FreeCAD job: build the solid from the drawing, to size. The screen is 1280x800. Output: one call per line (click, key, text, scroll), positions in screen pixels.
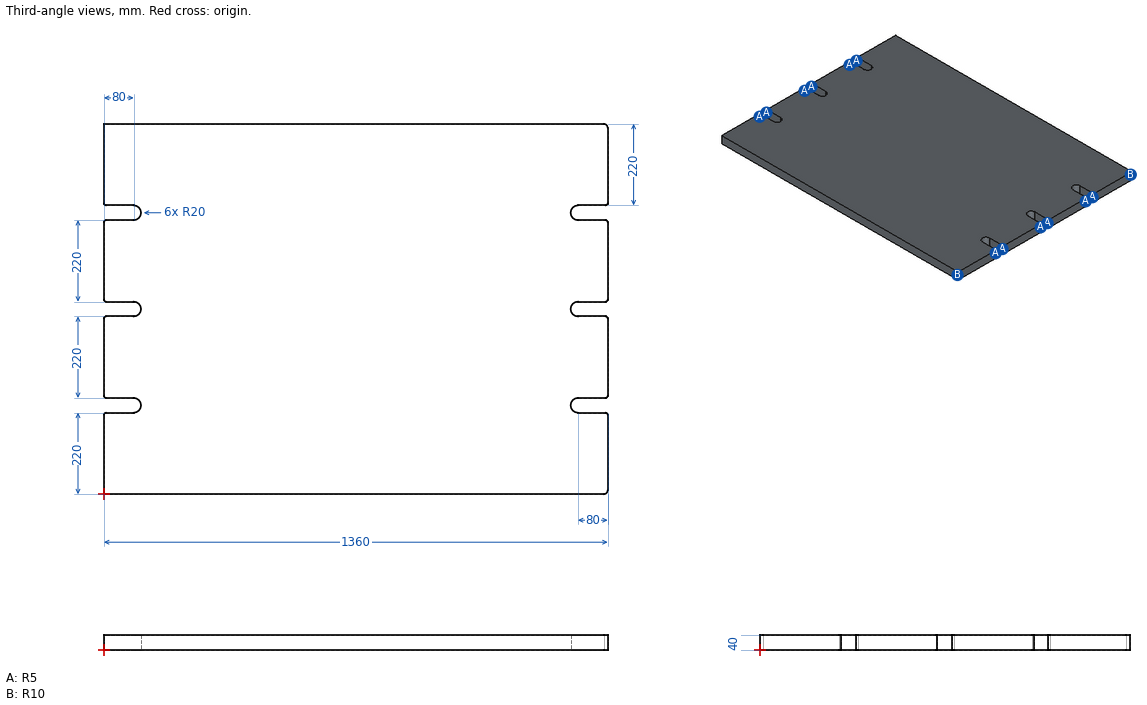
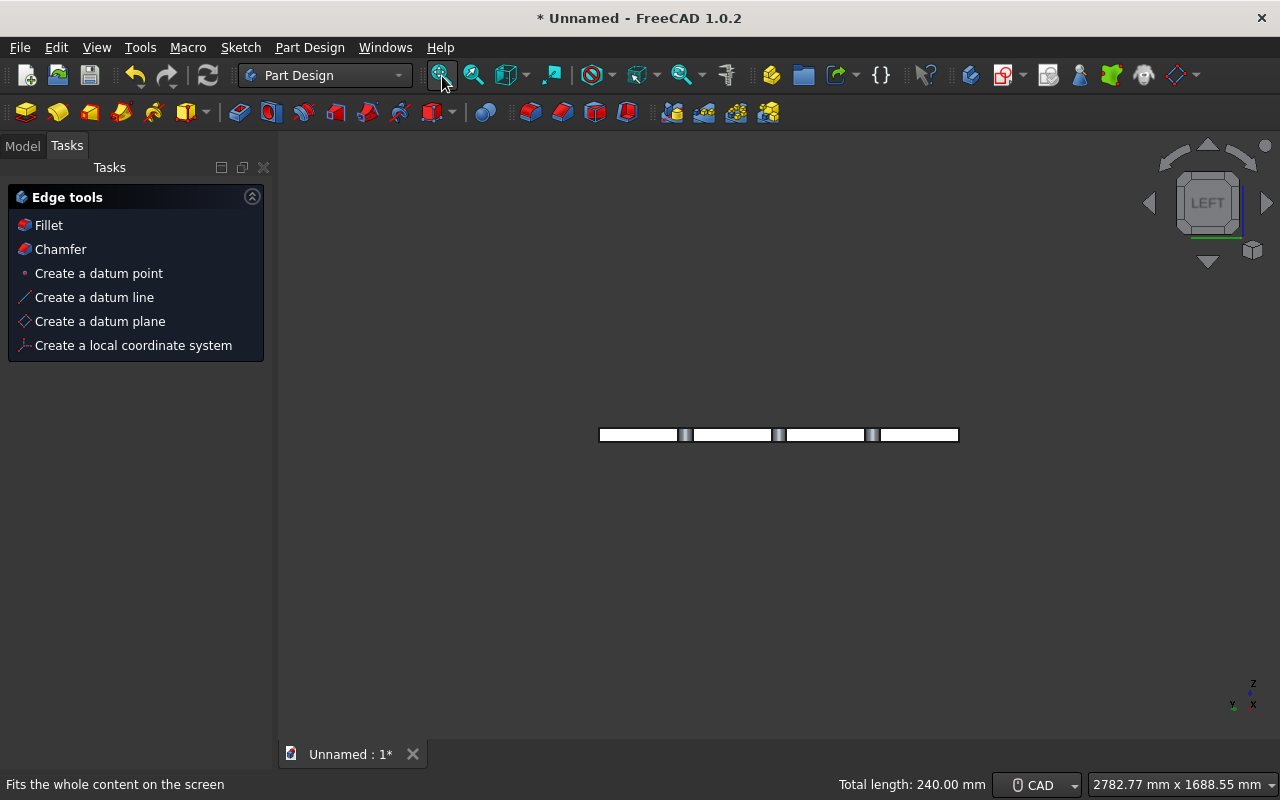
click(880, 434, ctrl)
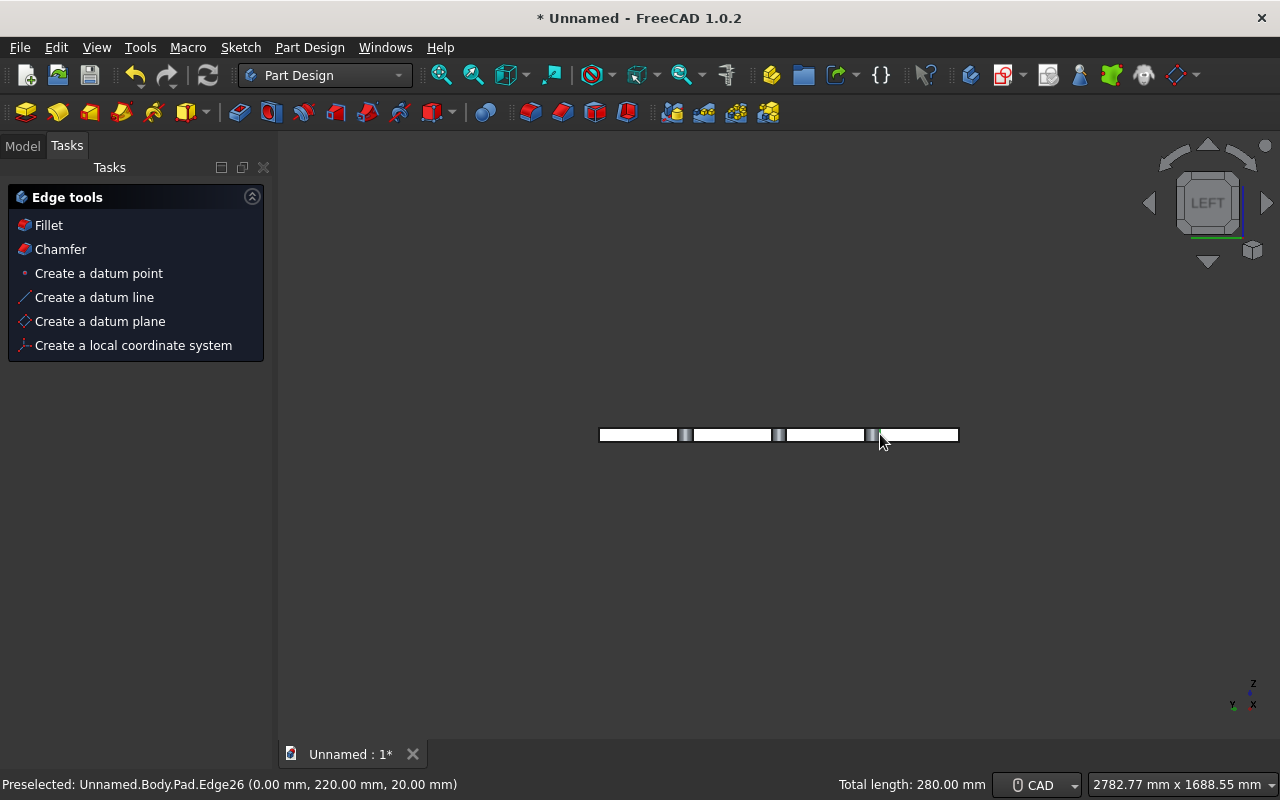
click(865, 434, ctrl)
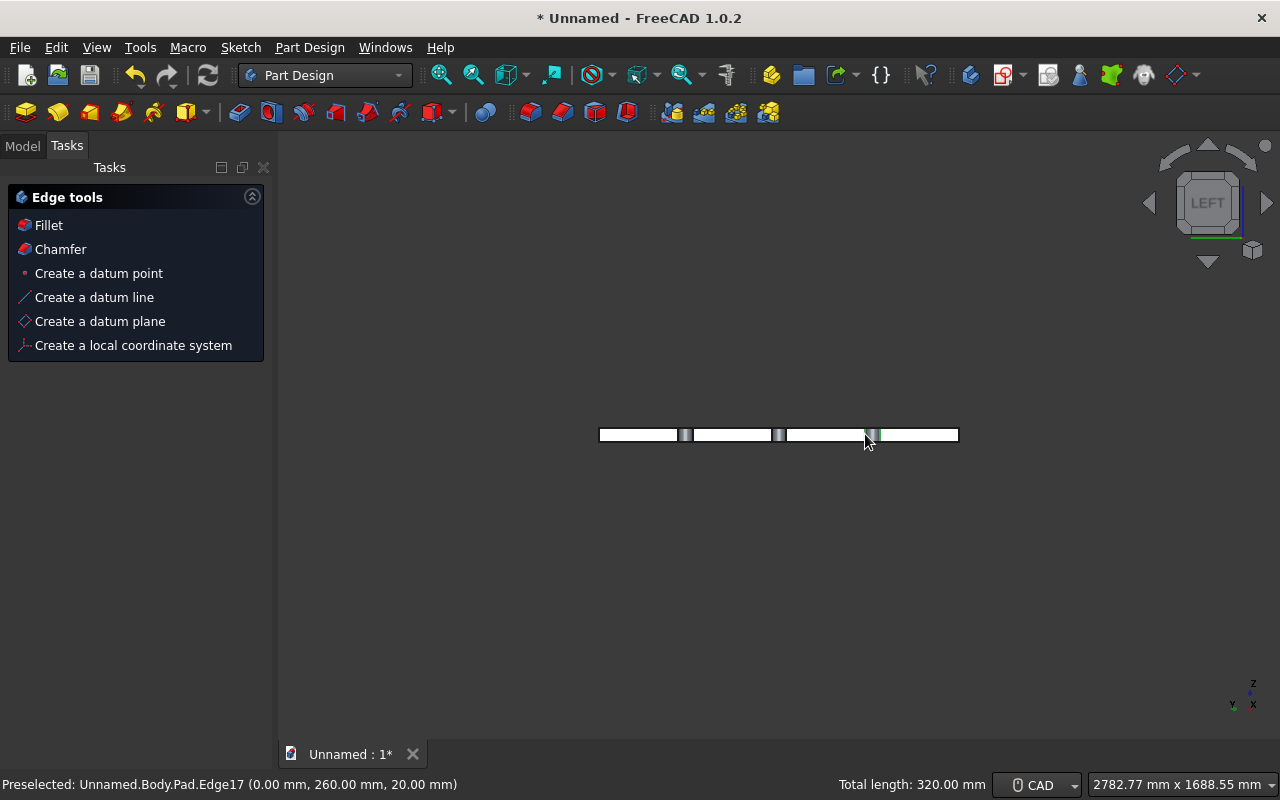
click(786, 434, ctrl)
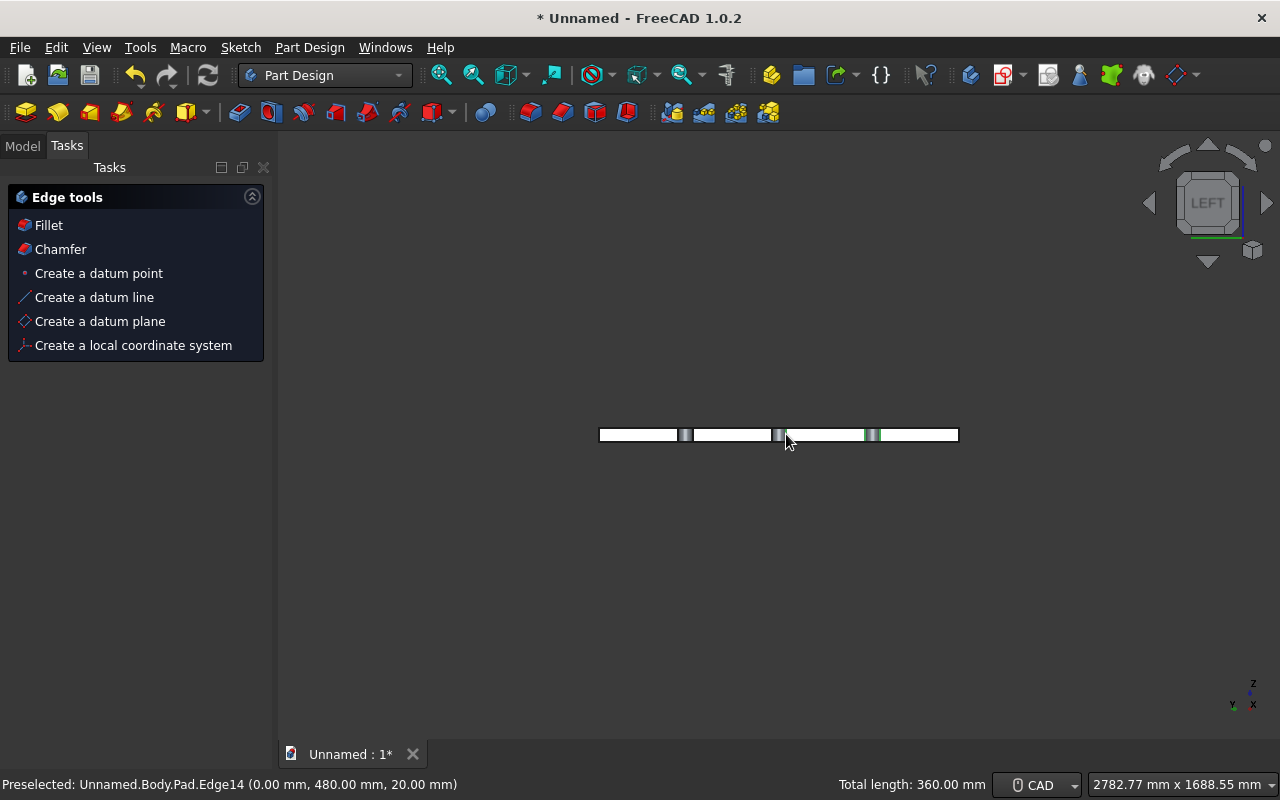
click(772, 434, ctrl)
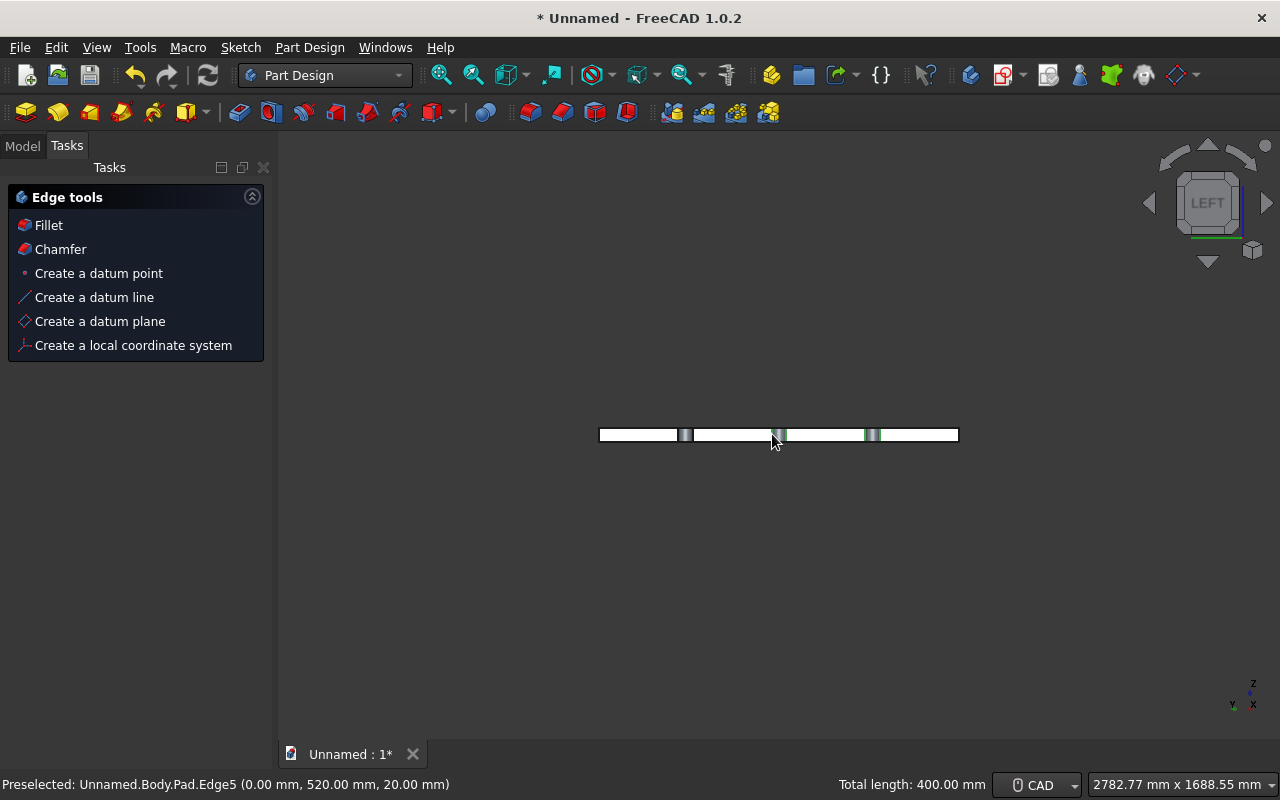
click(693, 434, ctrl)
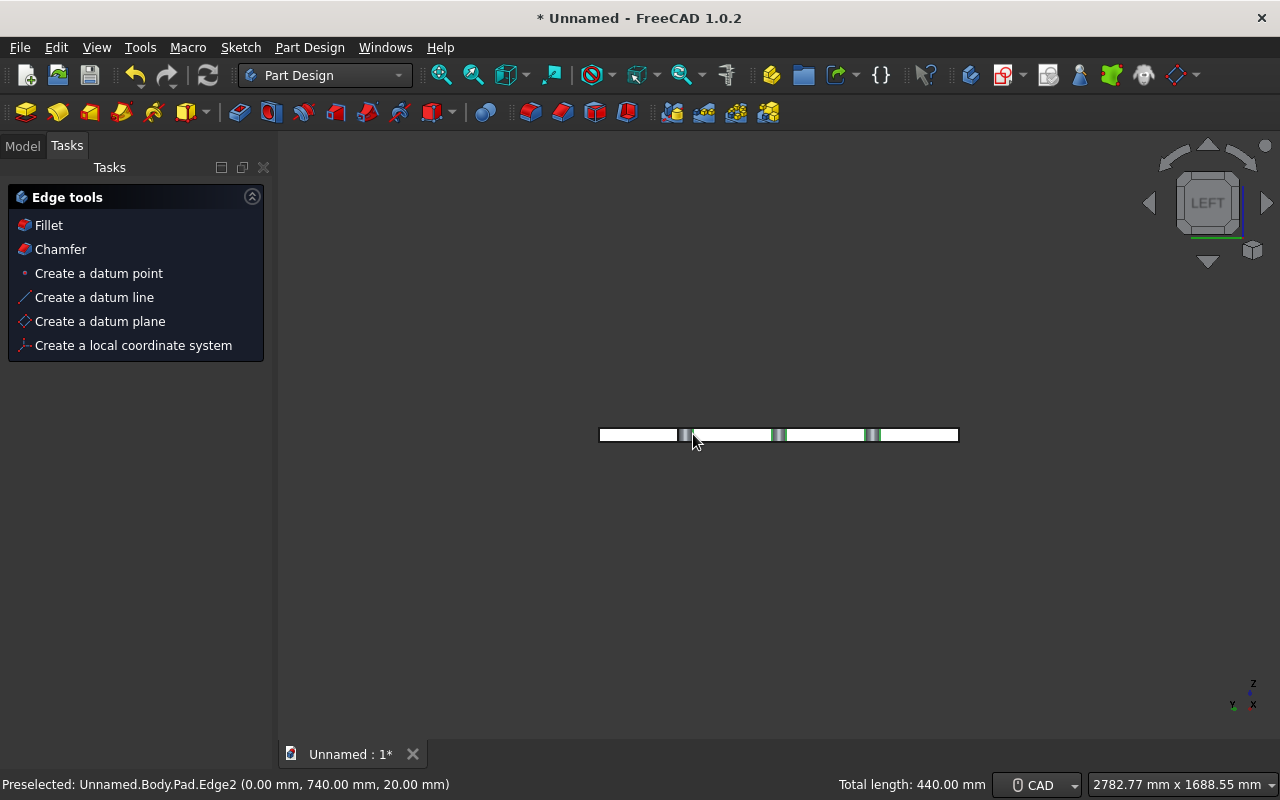
click(678, 434, ctrl)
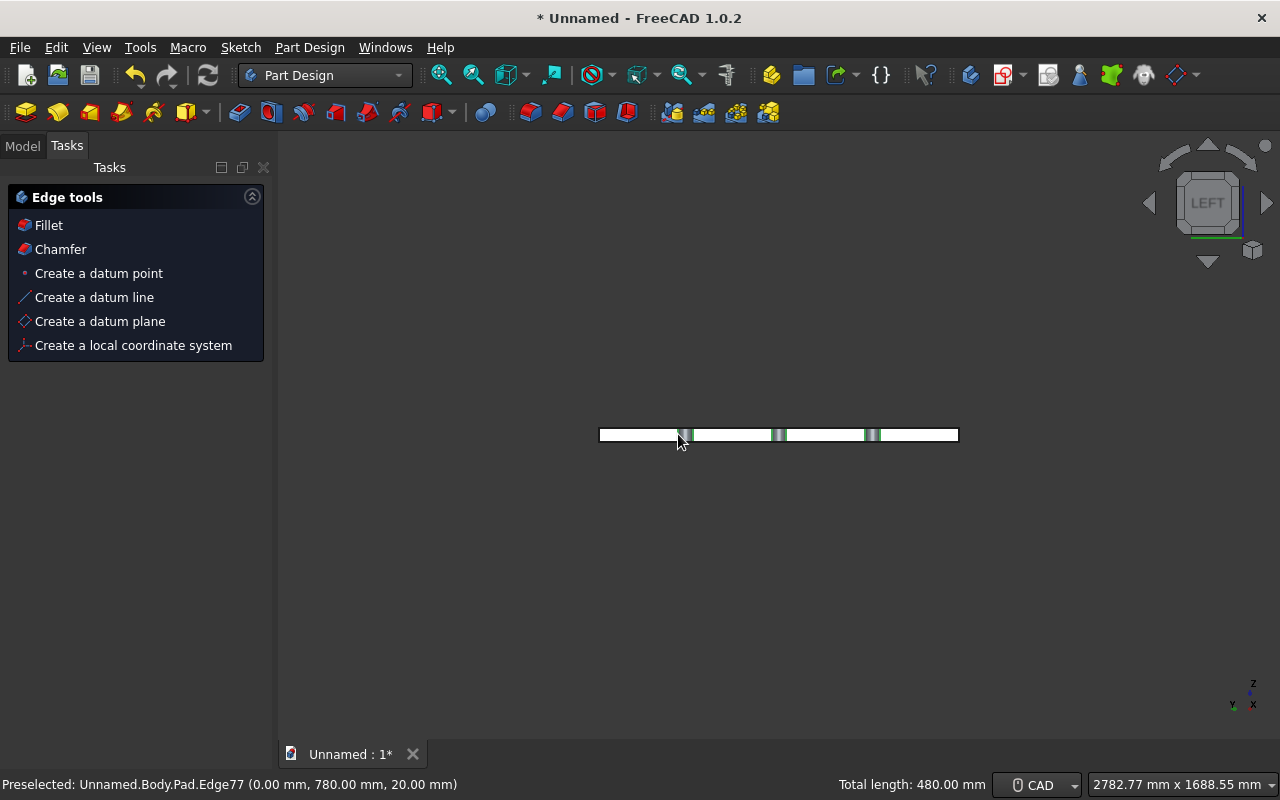
click(532, 112)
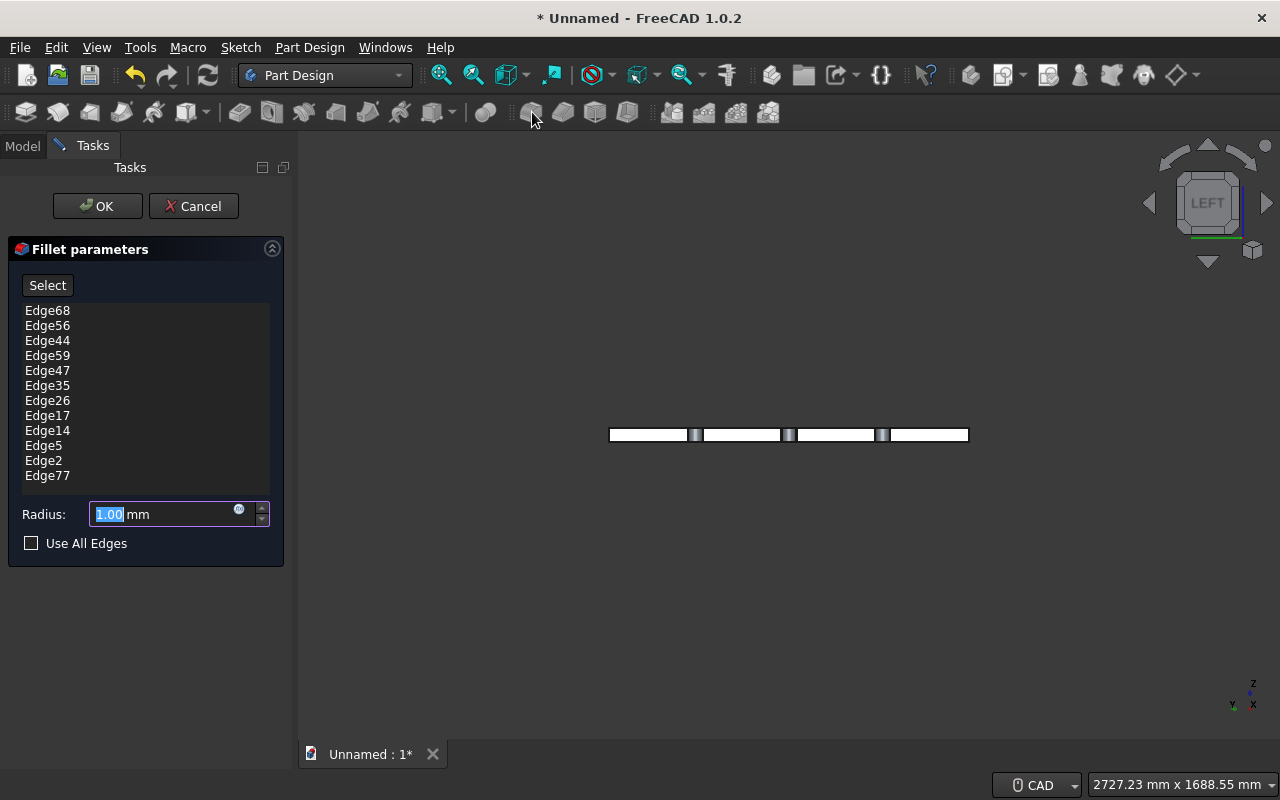
text(5)
key(Tab)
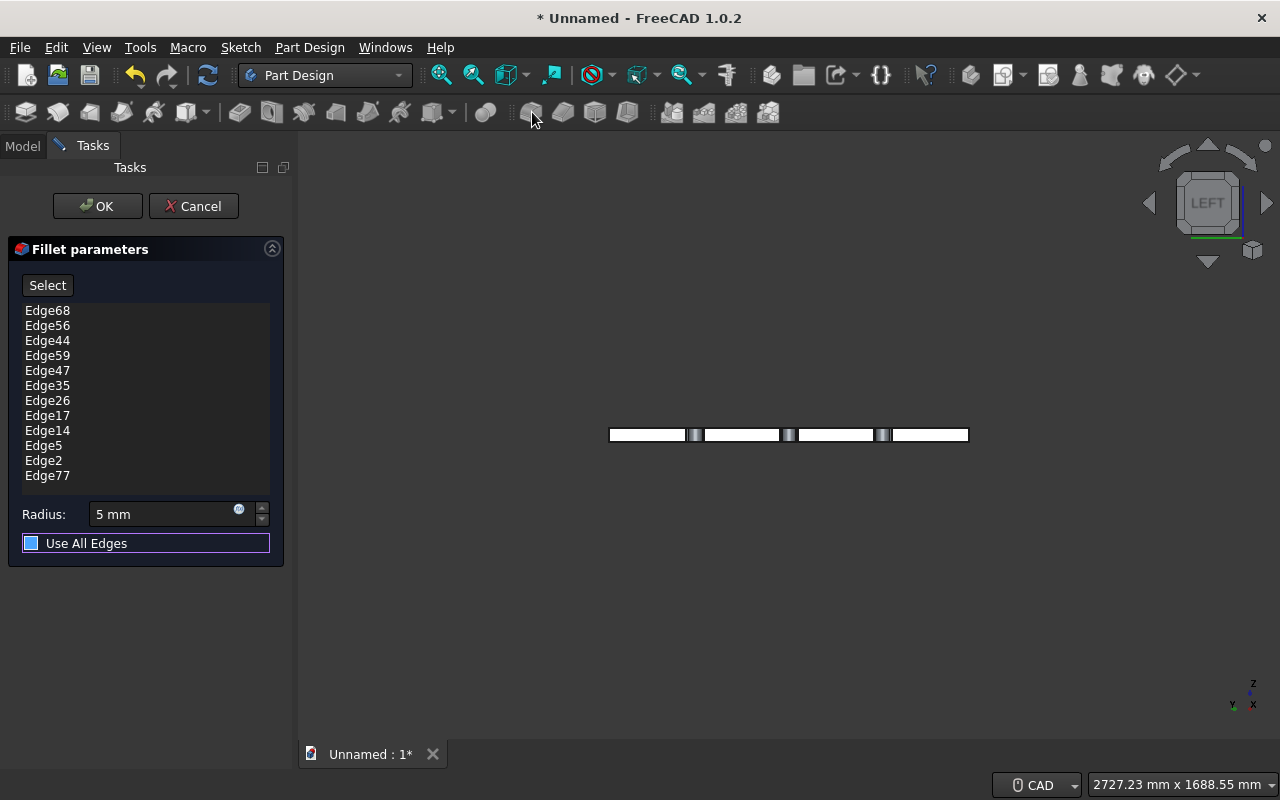
click(98, 206)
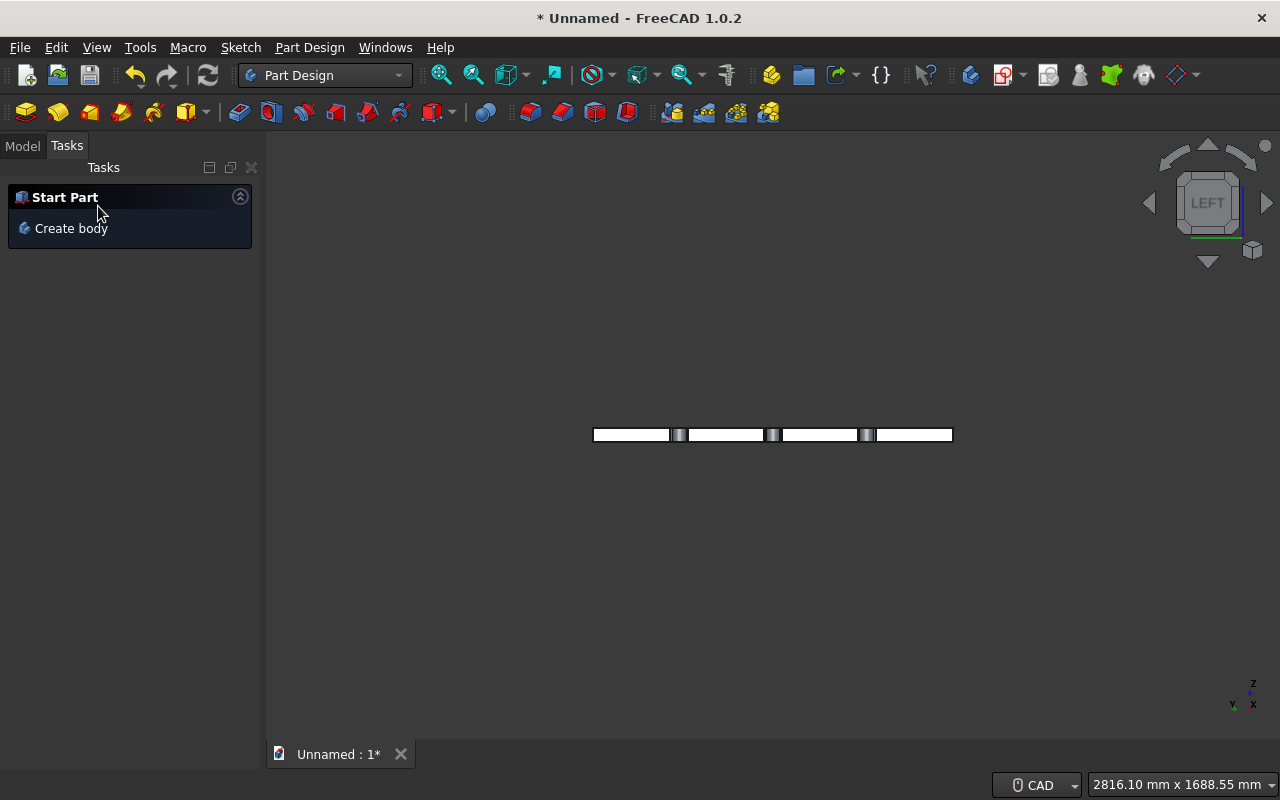
click(442, 76)